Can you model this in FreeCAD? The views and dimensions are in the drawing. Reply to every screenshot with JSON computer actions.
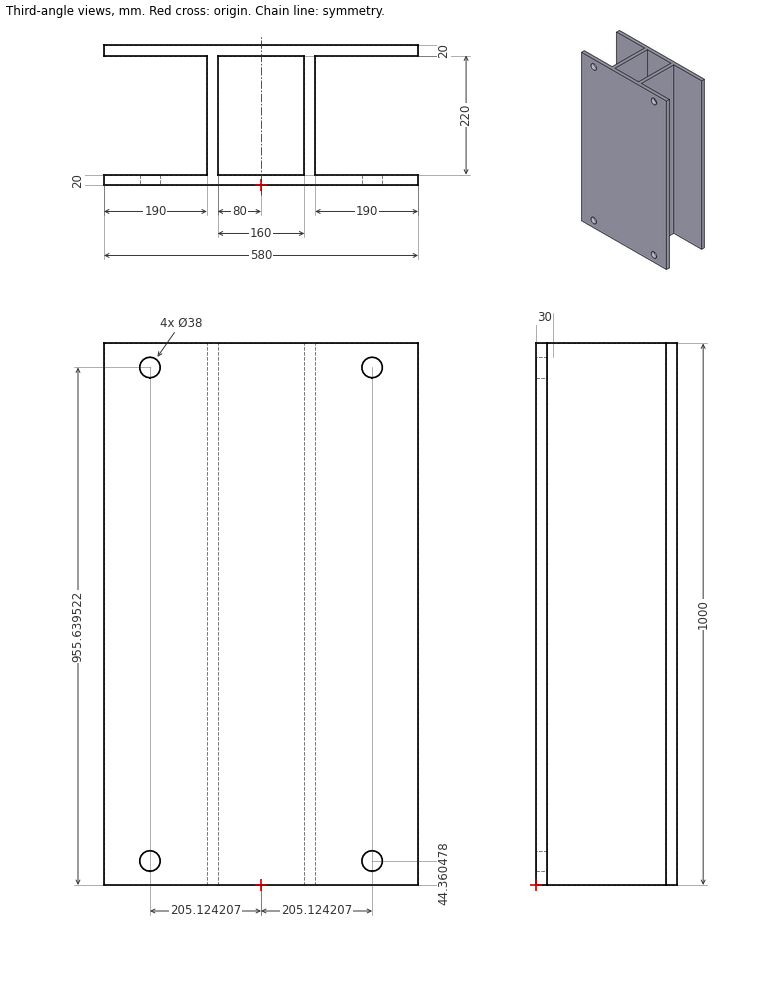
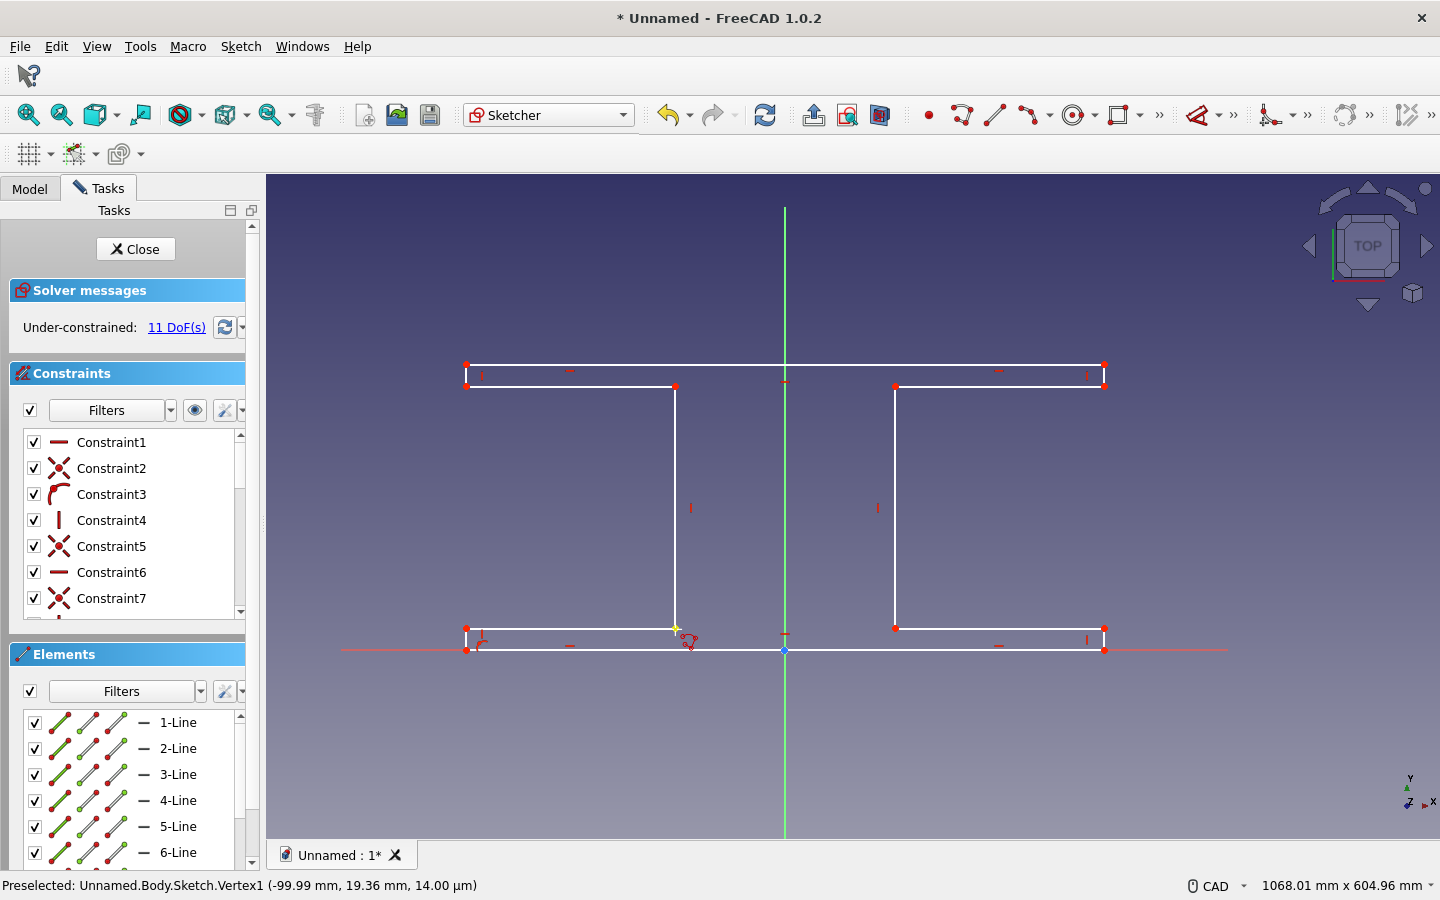
{"action": "key", "text": "g r"}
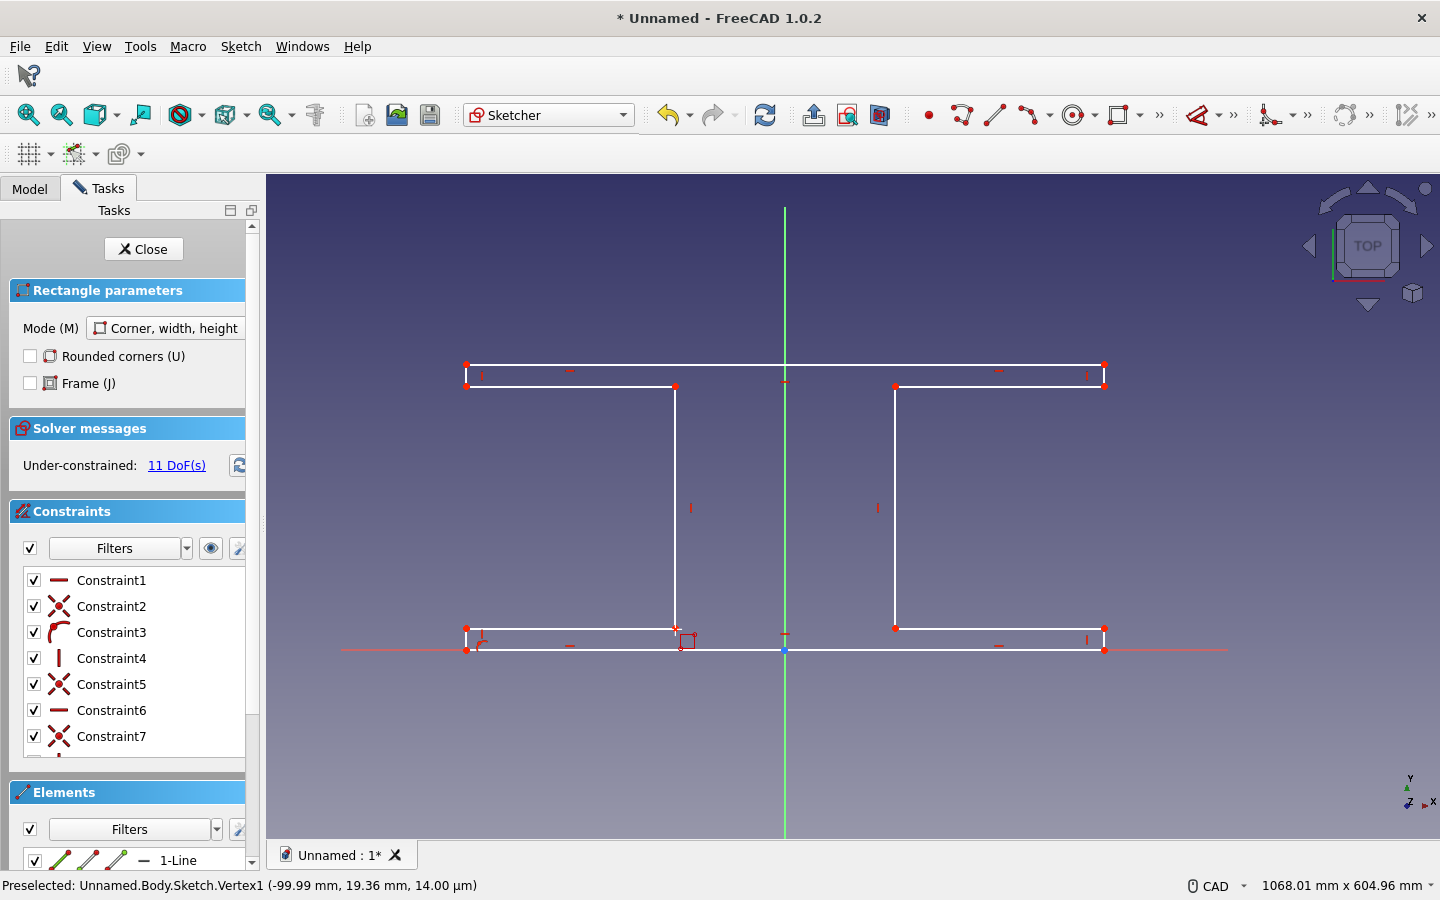
{"action": "left_click", "coordinate": [697, 386]}
{"action": "mouse_move", "coordinate": [873, 628]}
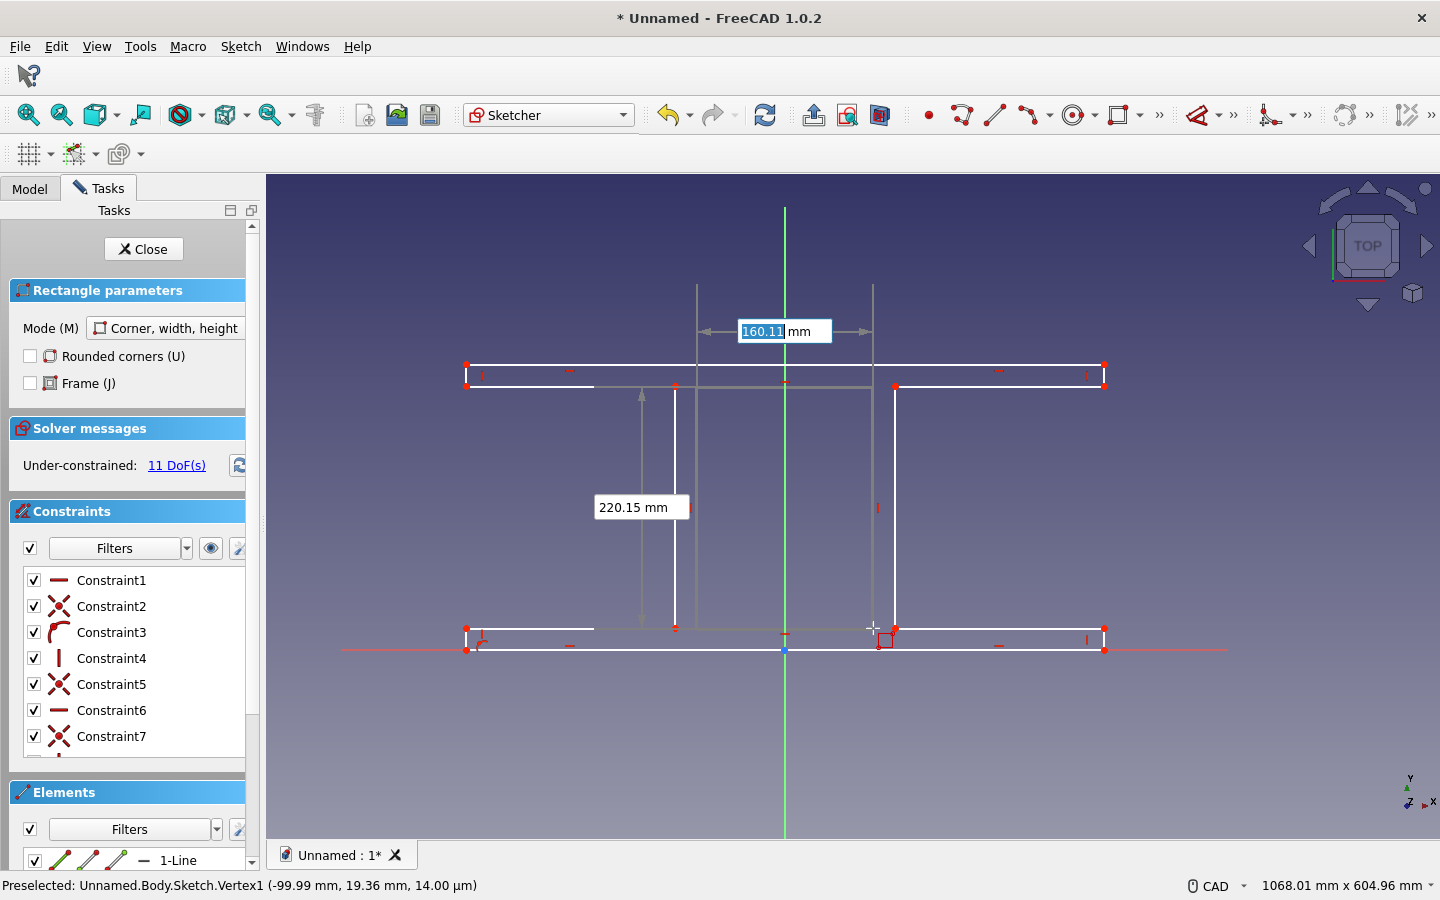
{"action": "type", "text": "160"}
{"action": "key", "text": "Tab"}
{"action": "type", "text": "220"}
{"action": "key", "text": "Return"}
{"action": "key", "text": "Escape"}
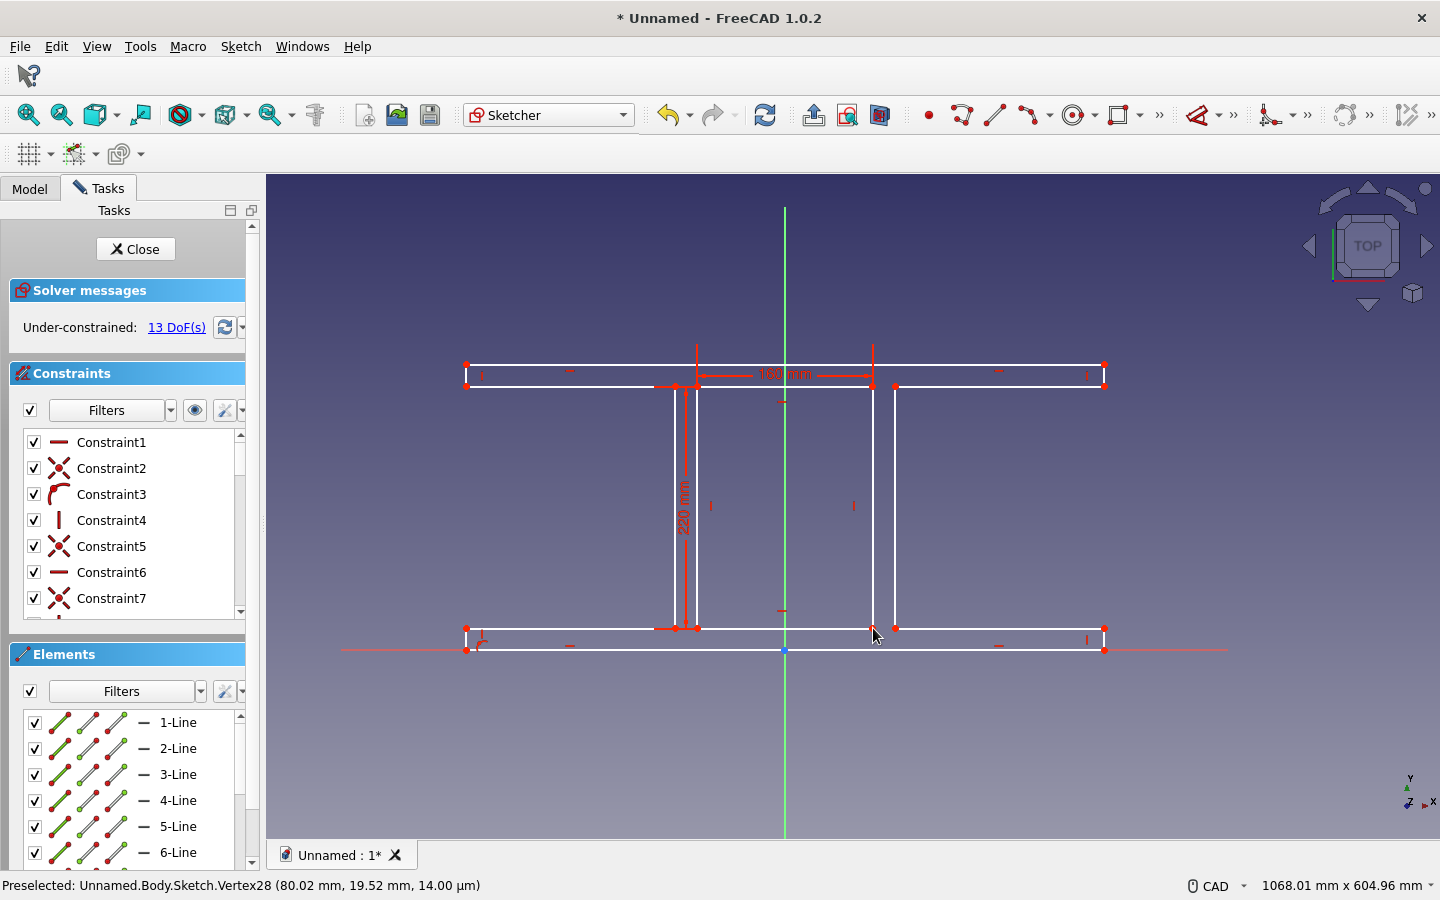
{"action": "left_click", "coordinate": [466, 629]}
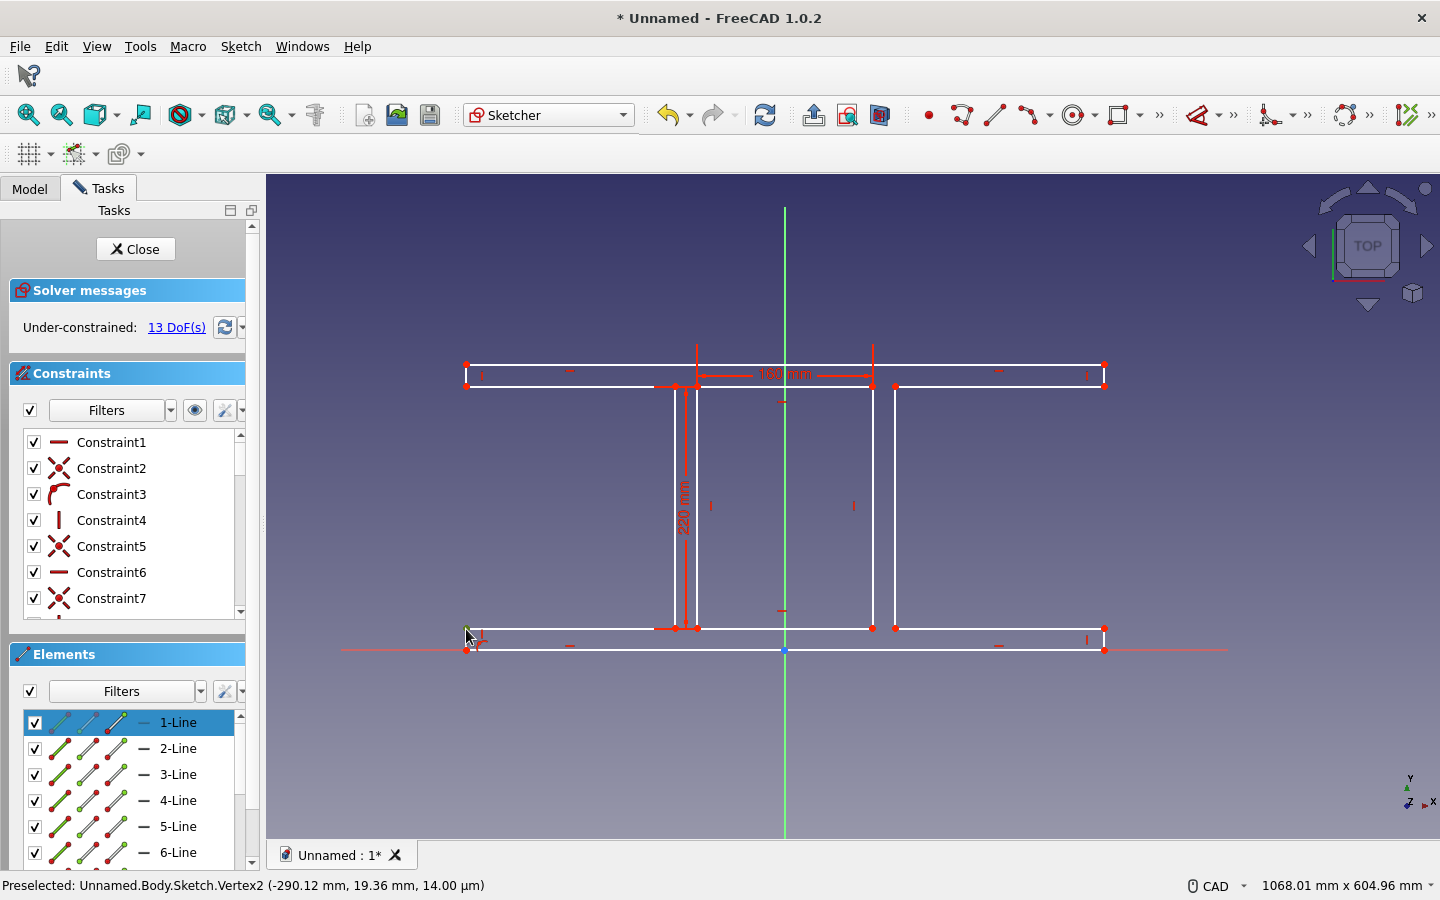
{"action": "left_click", "coordinate": [1104, 629]}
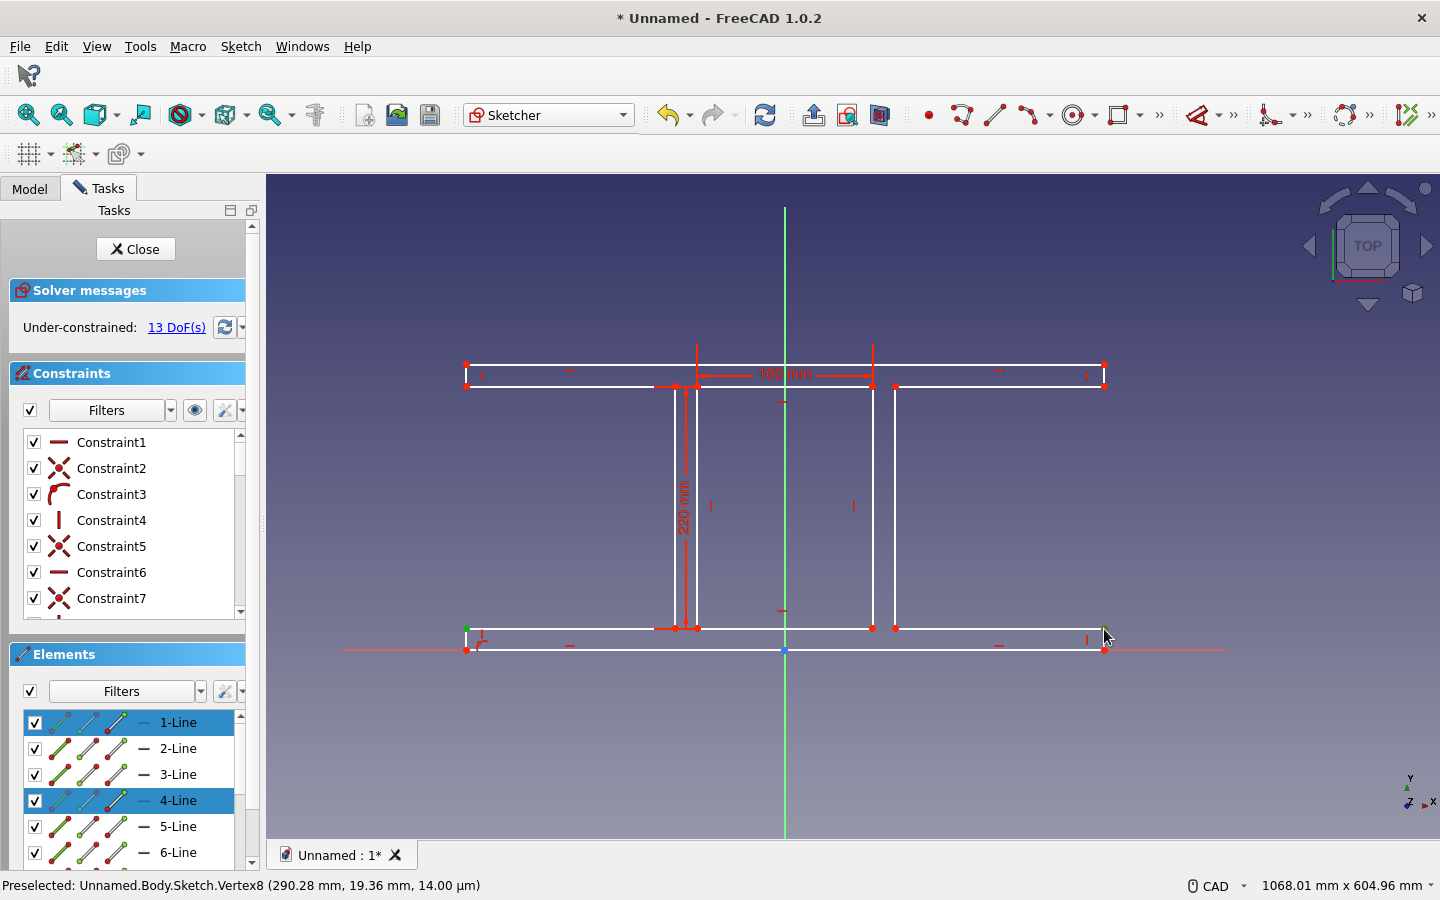
{"action": "left_click", "coordinate": [785, 768]}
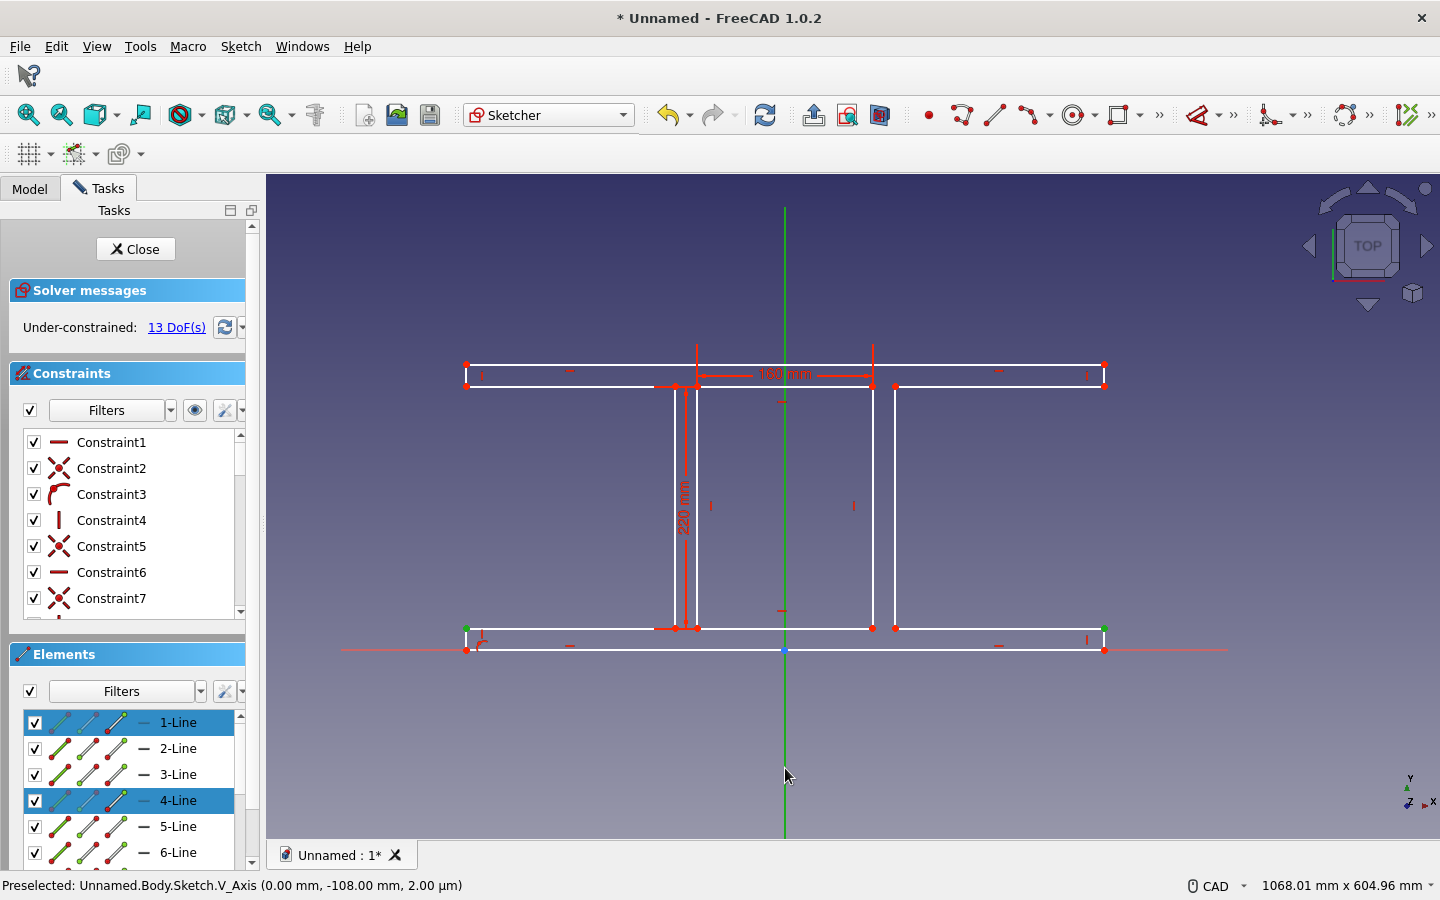
{"action": "key", "text": "s"}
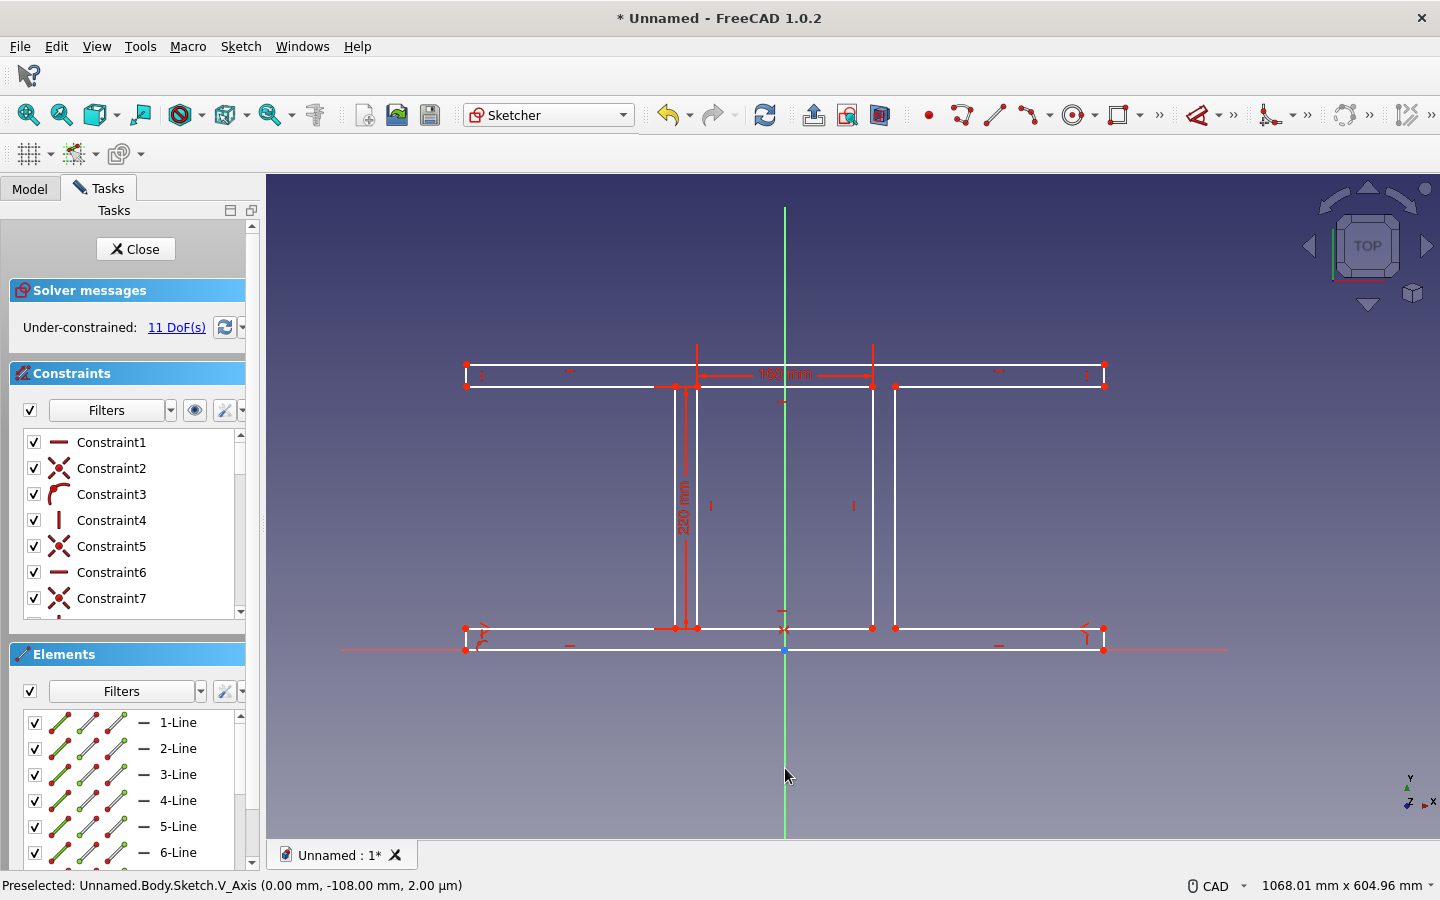
{"action": "left_click", "coordinate": [1104, 387]}